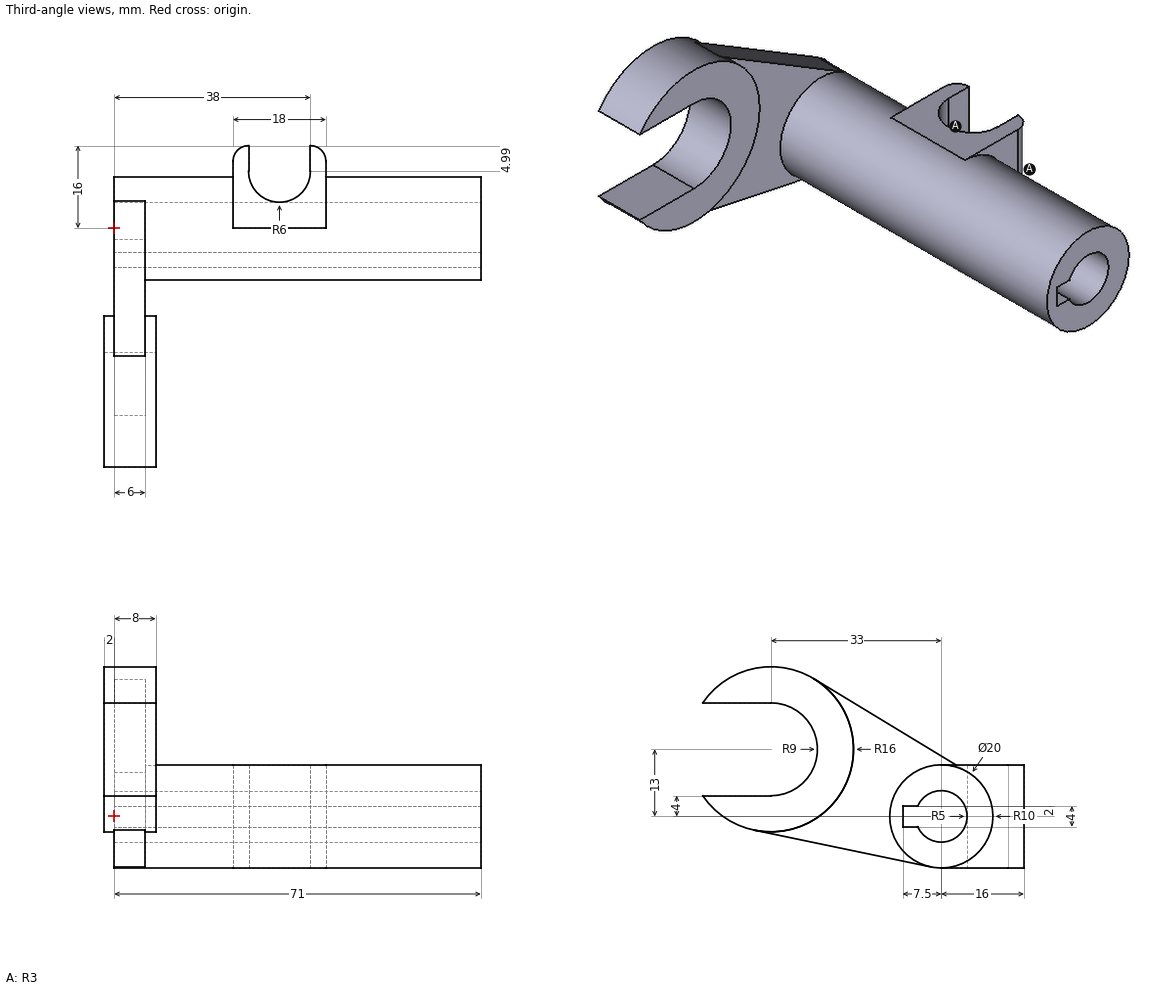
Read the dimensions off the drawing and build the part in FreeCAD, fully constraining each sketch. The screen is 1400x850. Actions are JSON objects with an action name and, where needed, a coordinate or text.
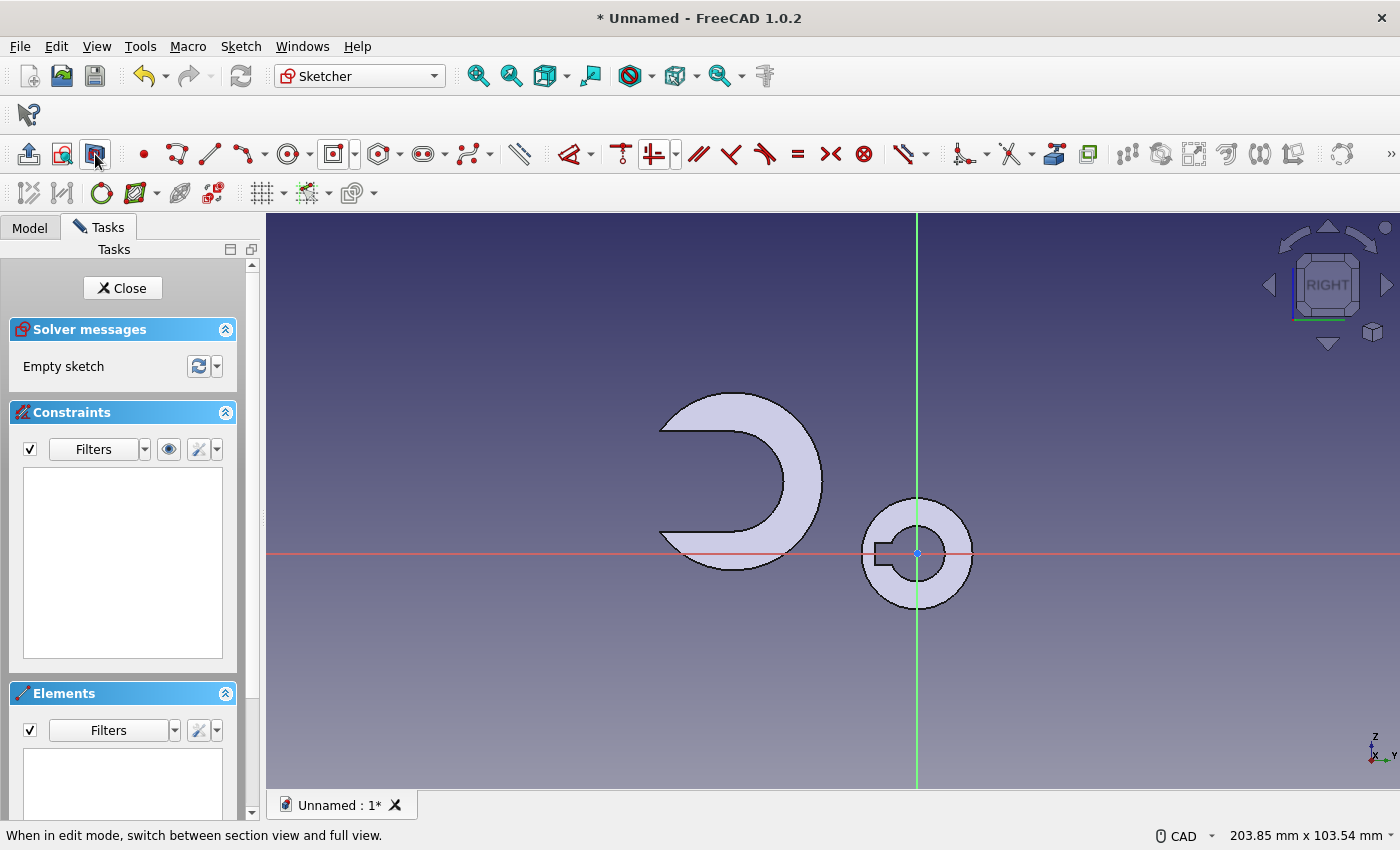
{"action": "scroll", "coordinate": [911, 514], "scroll_direction": "up", "scroll_amount": 3}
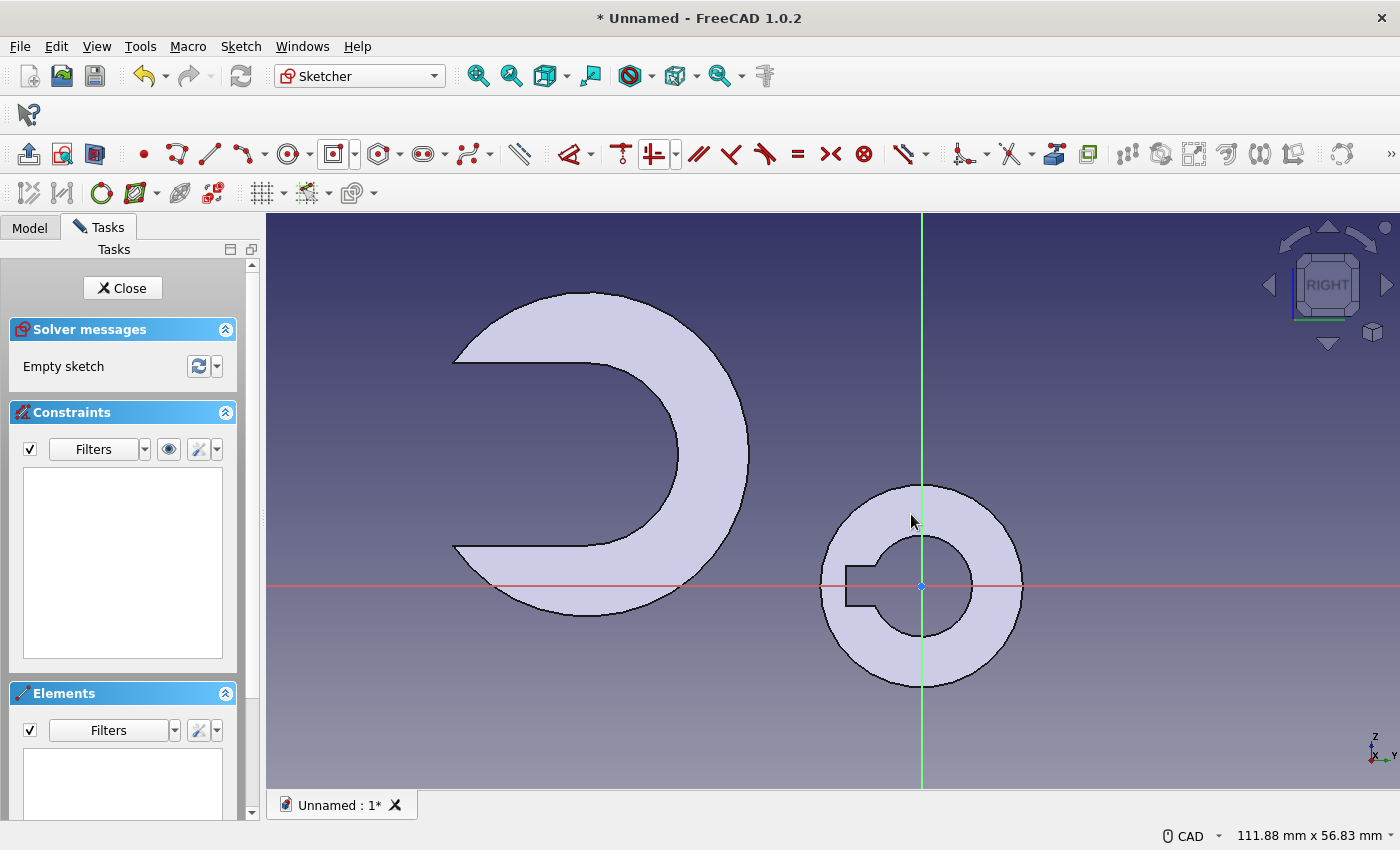
{"action": "key", "text": "g l"}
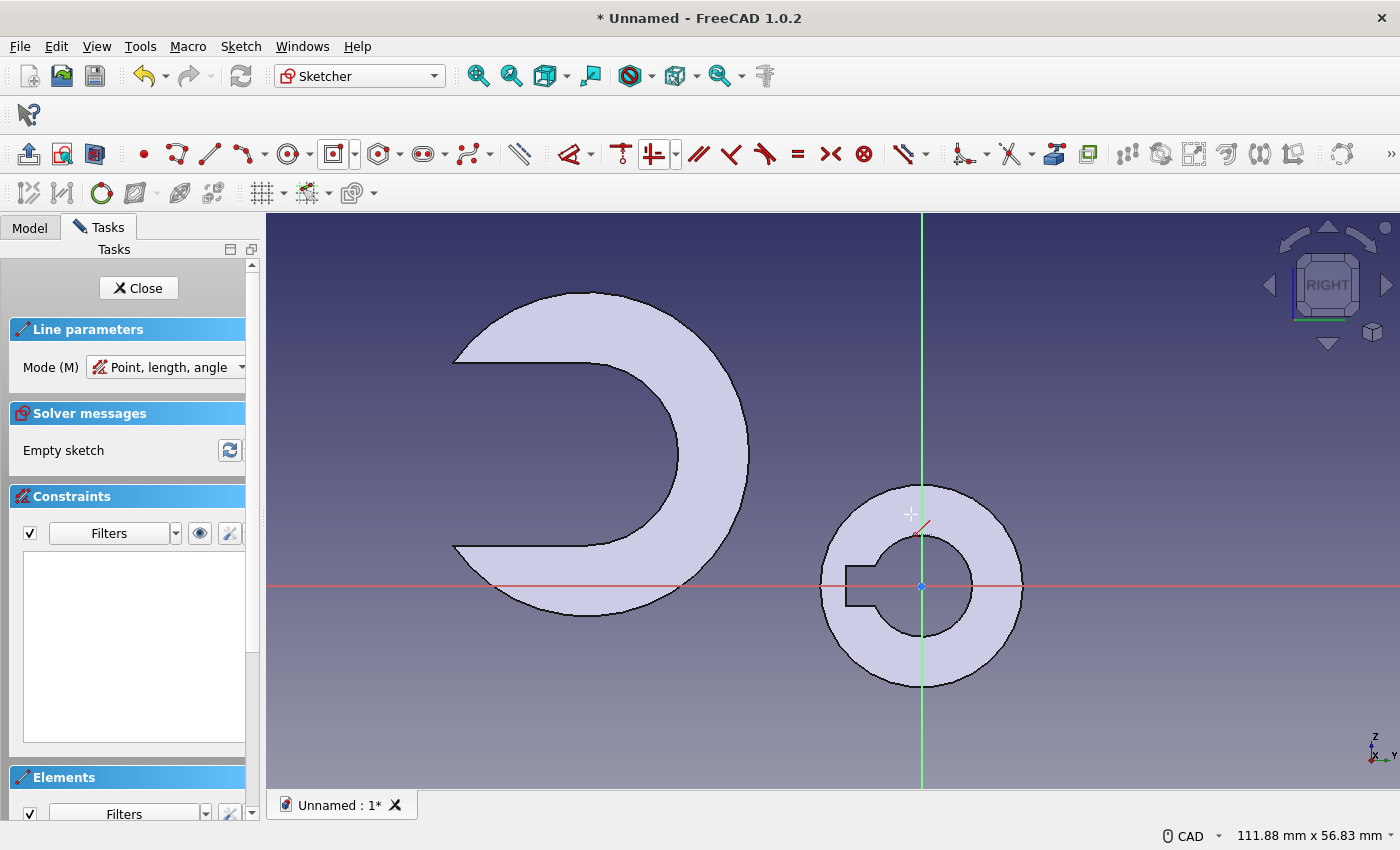
{"action": "left_click", "coordinate": [671, 316]}
{"action": "left_click", "coordinate": [974, 499]}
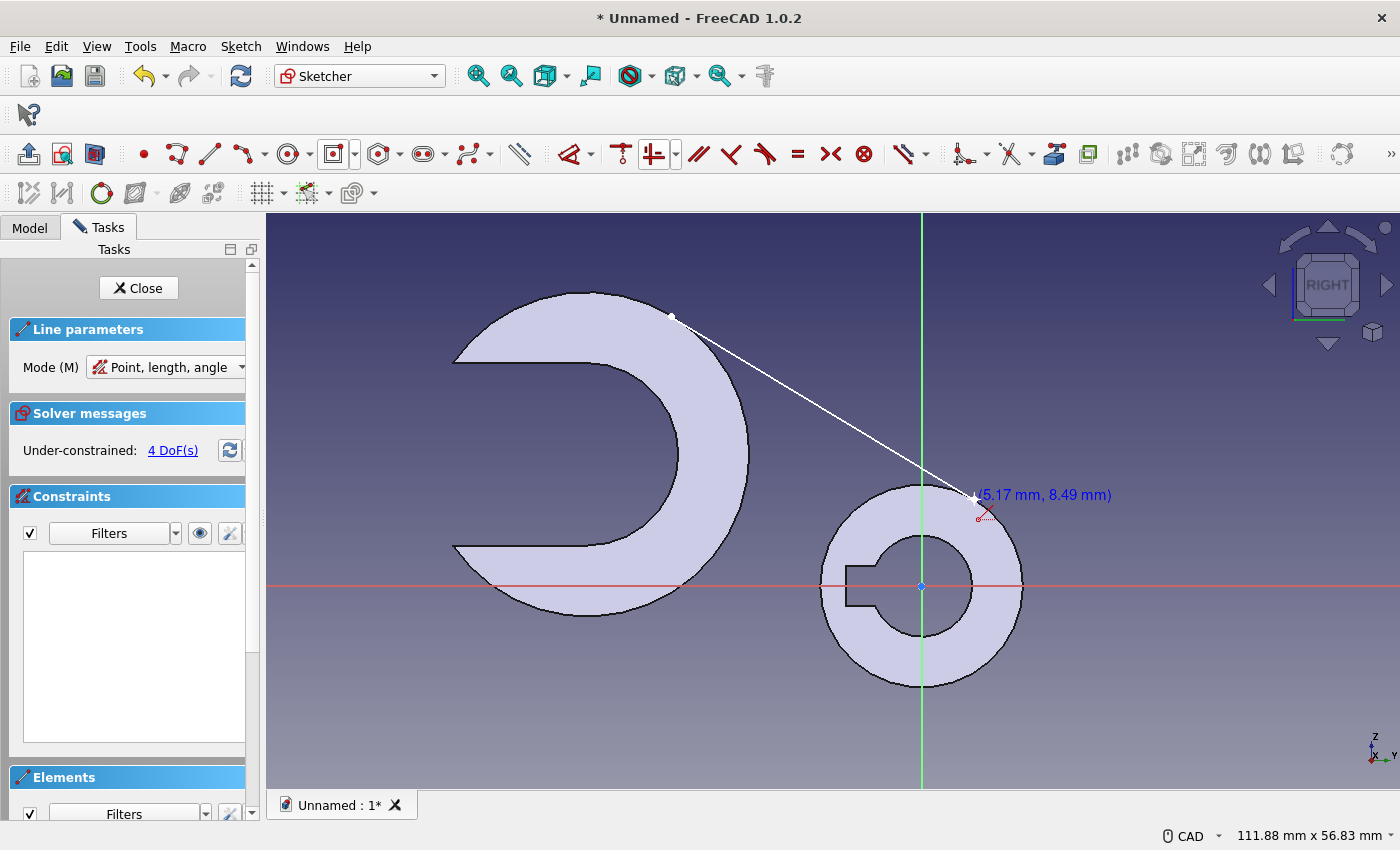
{"action": "left_click", "coordinate": [901, 685]}
{"action": "left_click", "coordinate": [554, 613]}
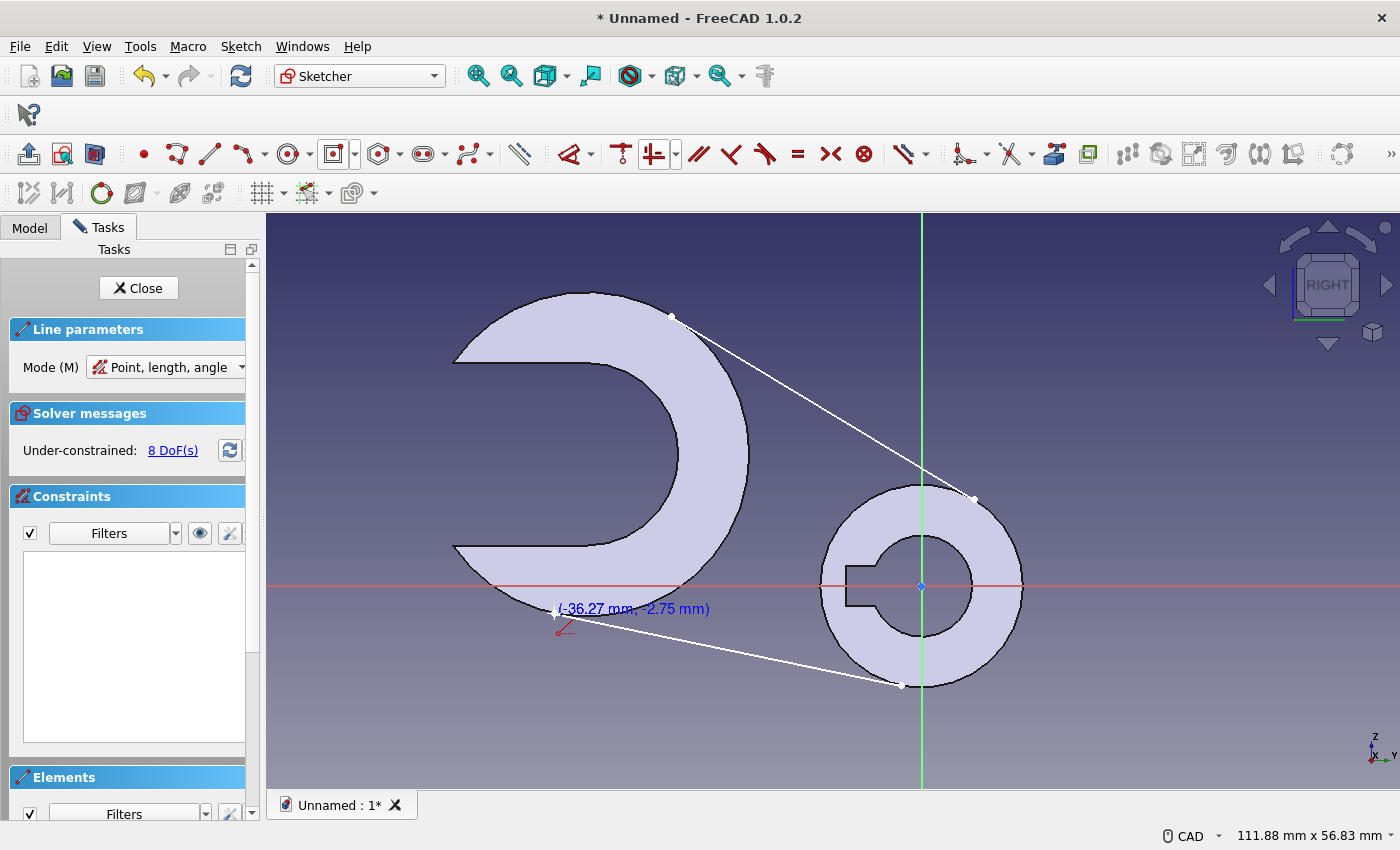
{"action": "left_click", "coordinate": [242, 154]}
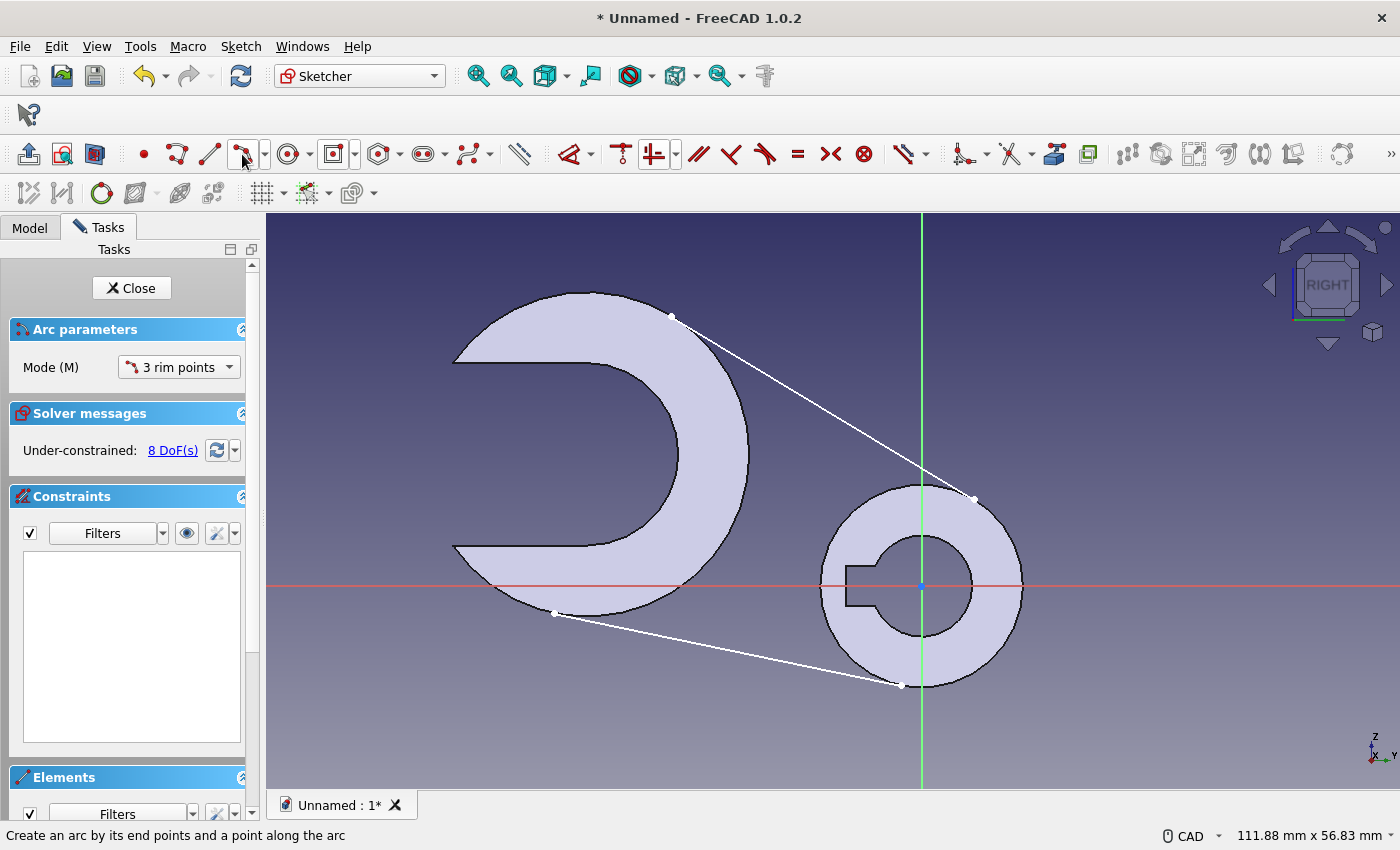
{"action": "left_click", "coordinate": [974, 500]}
{"action": "left_click", "coordinate": [901, 686]}
{"action": "left_click", "coordinate": [827, 549]}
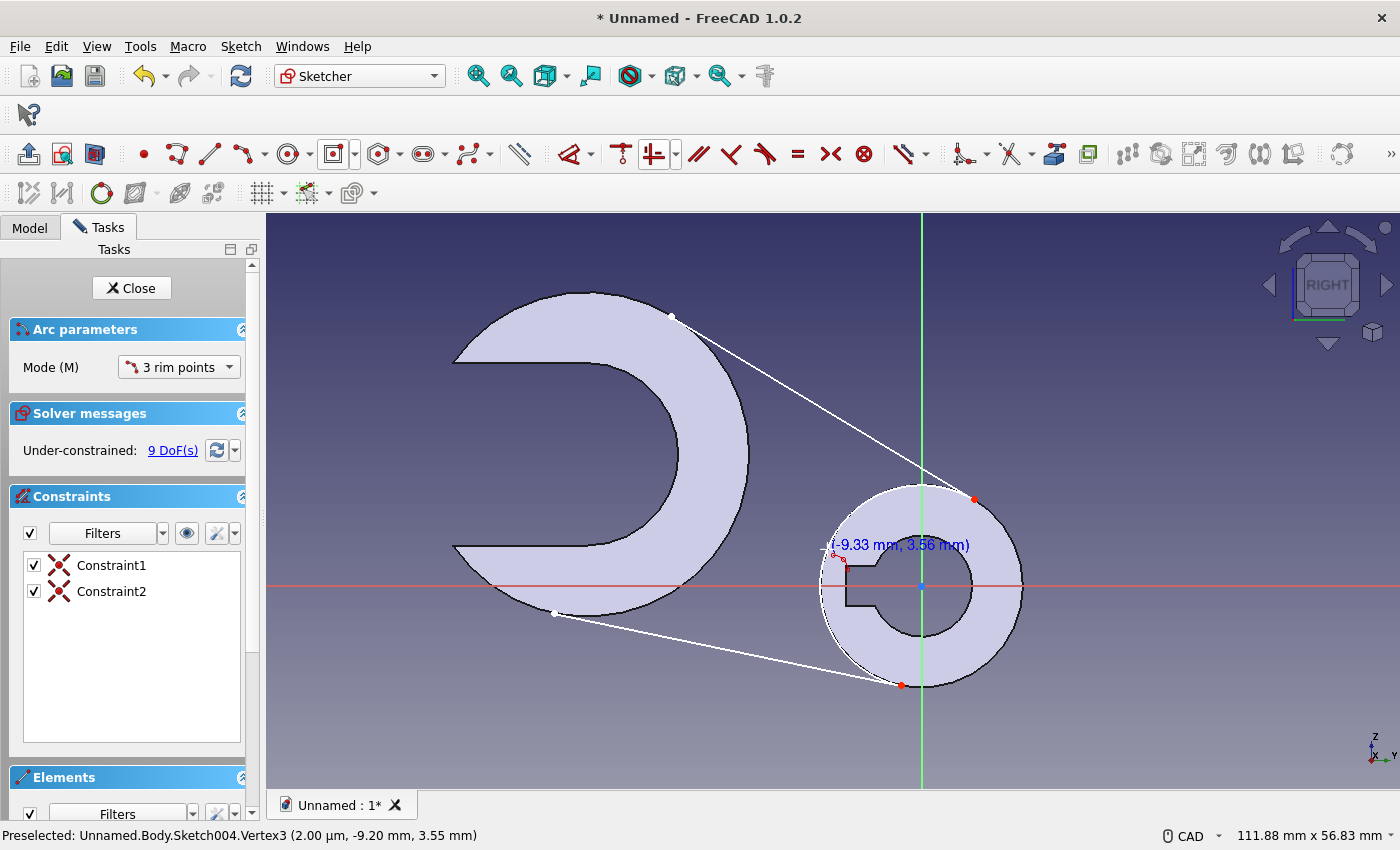
{"action": "left_click", "coordinate": [554, 614]}
{"action": "left_click", "coordinate": [671, 317]}
{"action": "left_click", "coordinate": [738, 514]}
{"action": "key", "text": "Escape"}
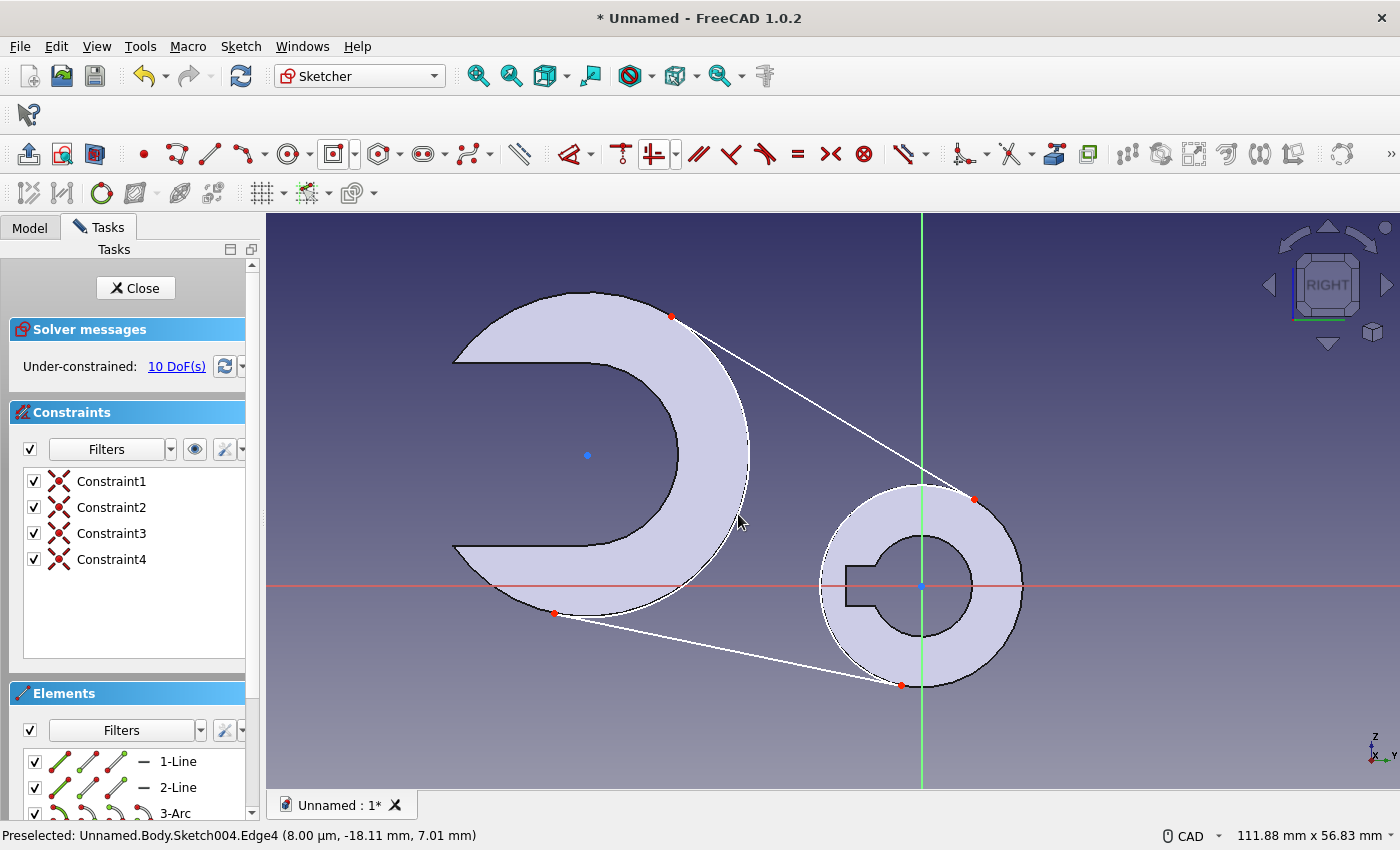
{"action": "left_click", "coordinate": [762, 372]}